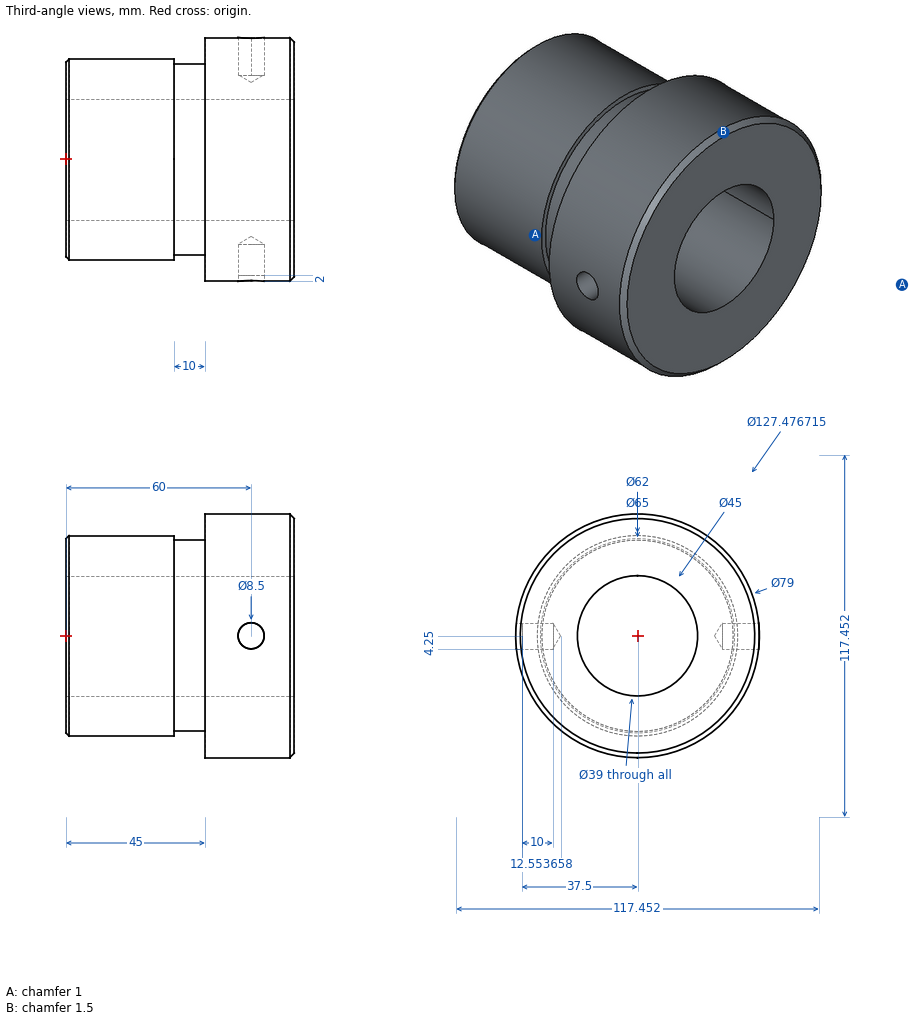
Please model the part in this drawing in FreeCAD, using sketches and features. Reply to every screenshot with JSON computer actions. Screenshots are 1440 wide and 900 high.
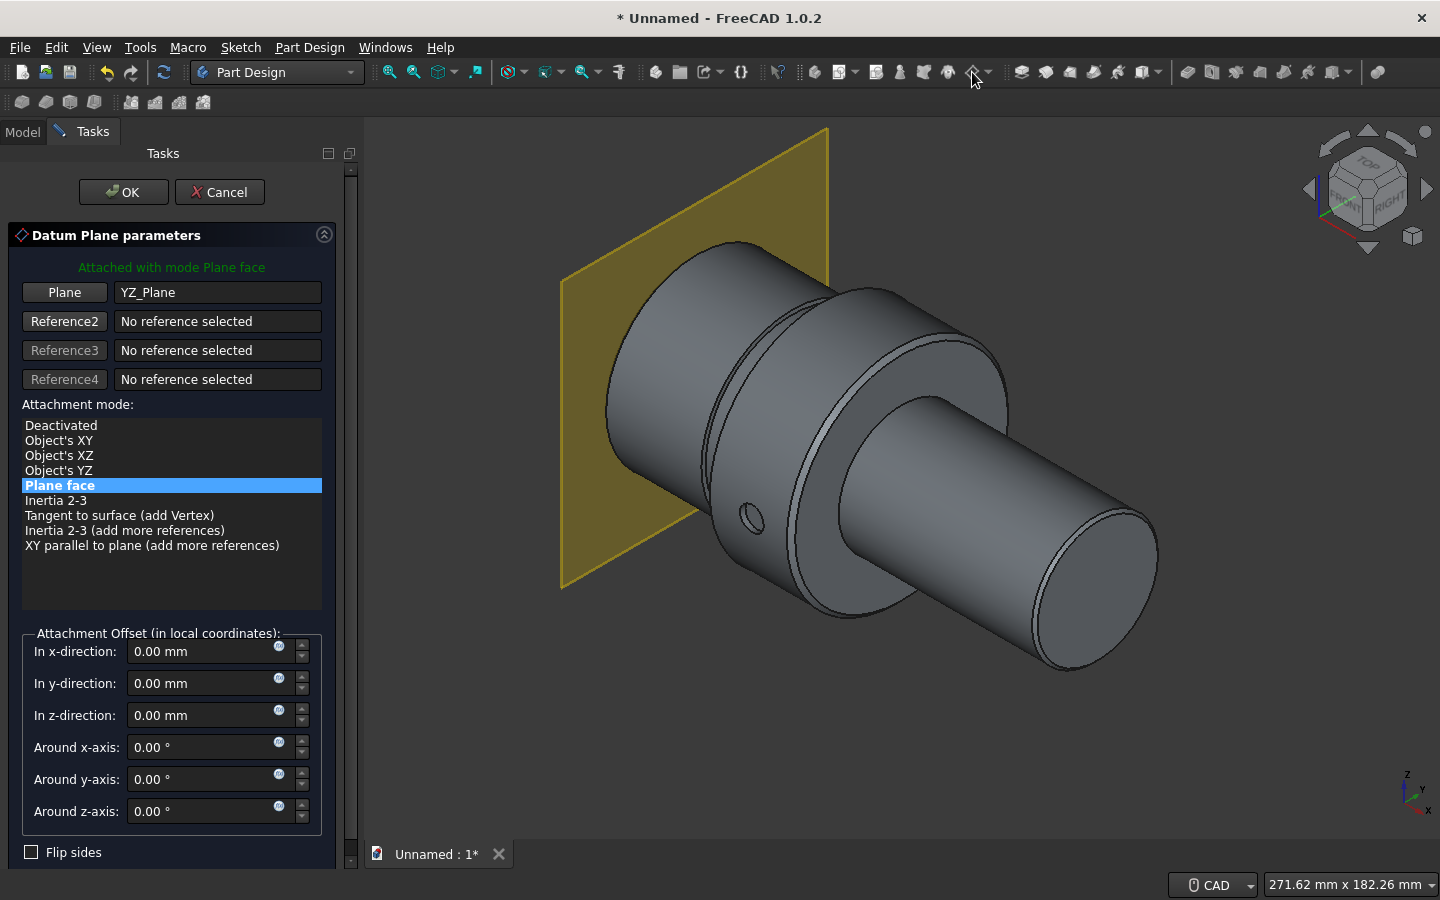
{"action": "triple_click", "coordinate": [210, 715]}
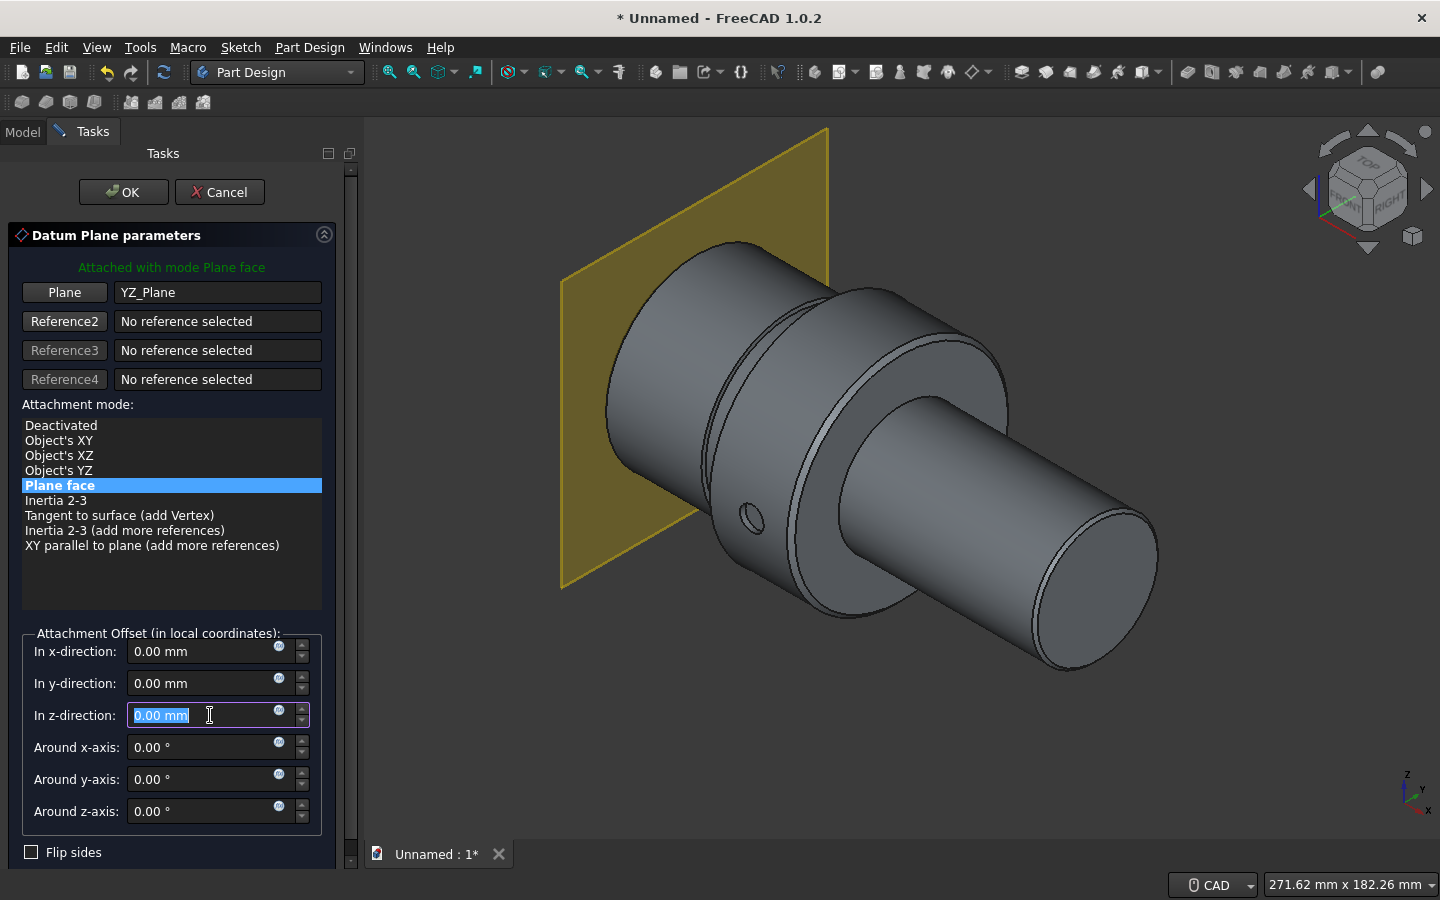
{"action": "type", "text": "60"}
{"action": "key", "text": "Tab"}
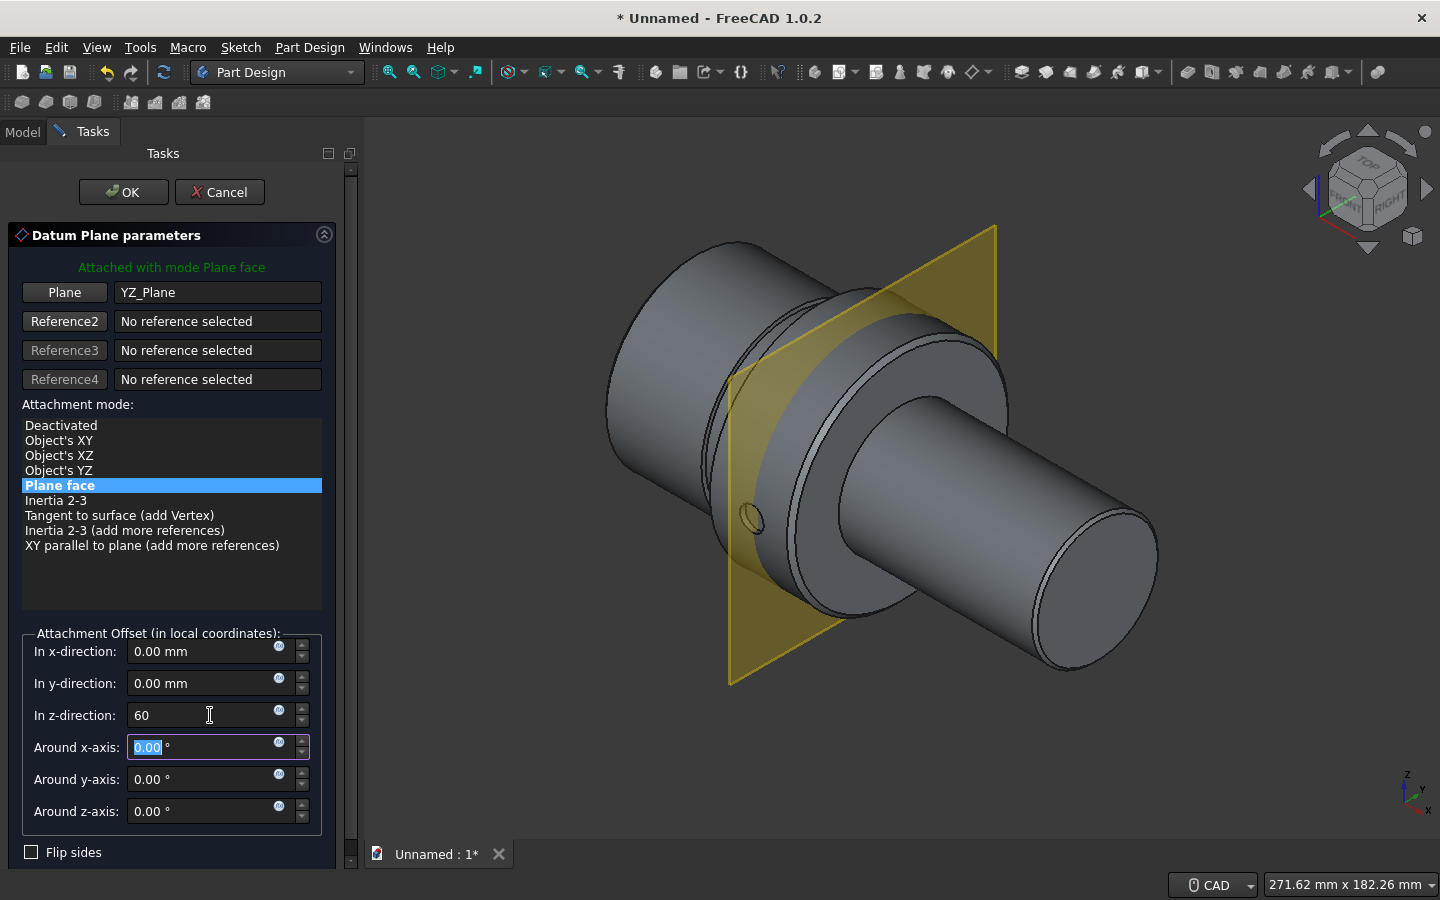
{"action": "left_click", "coordinate": [124, 192]}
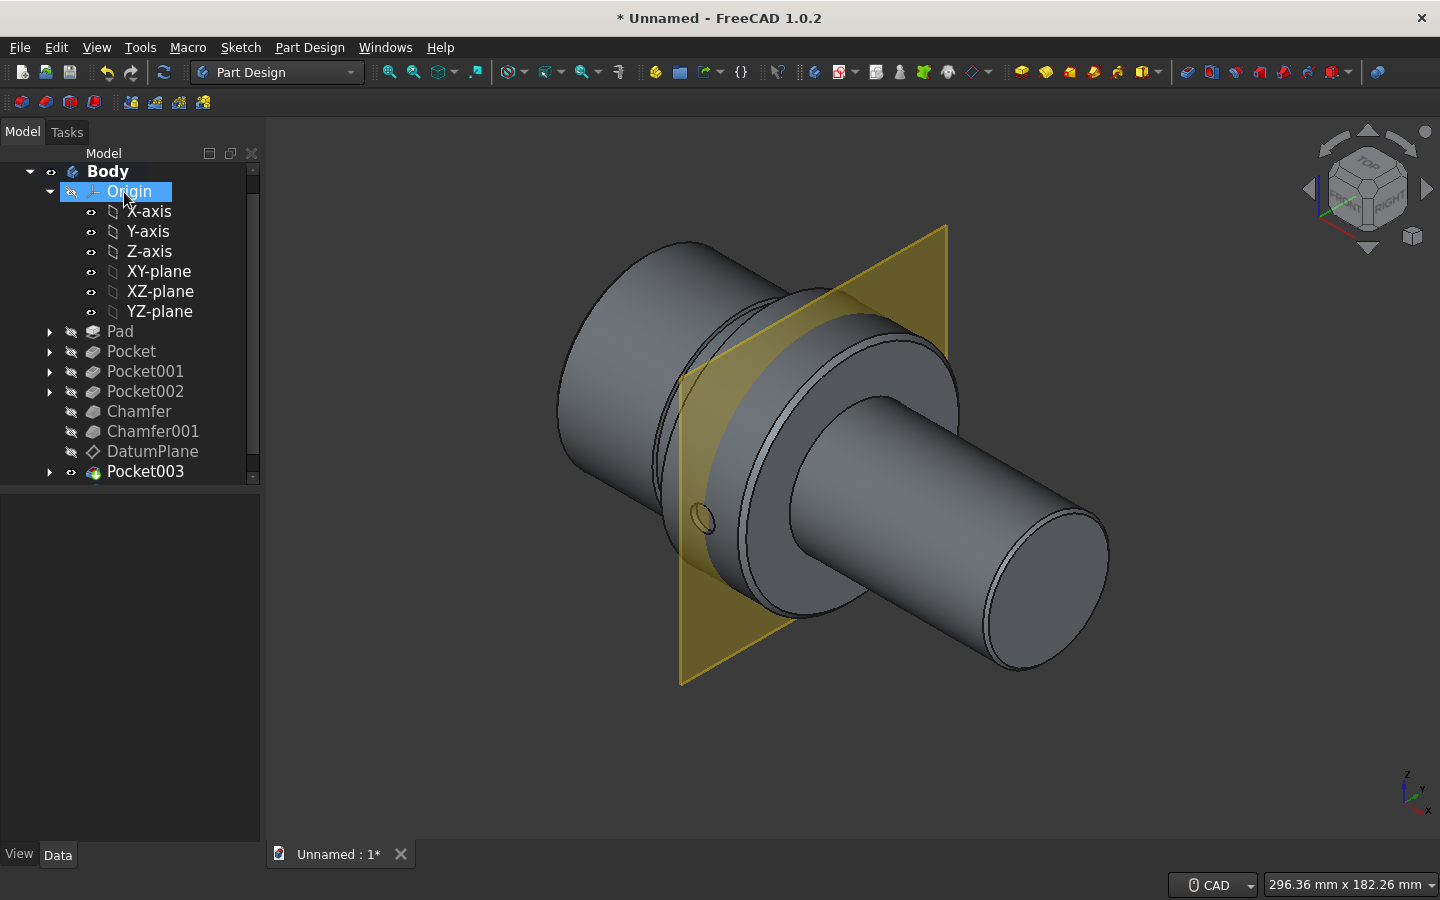
{"action": "scroll", "coordinate": [120, 327], "scroll_direction": "down", "scroll_amount": 3}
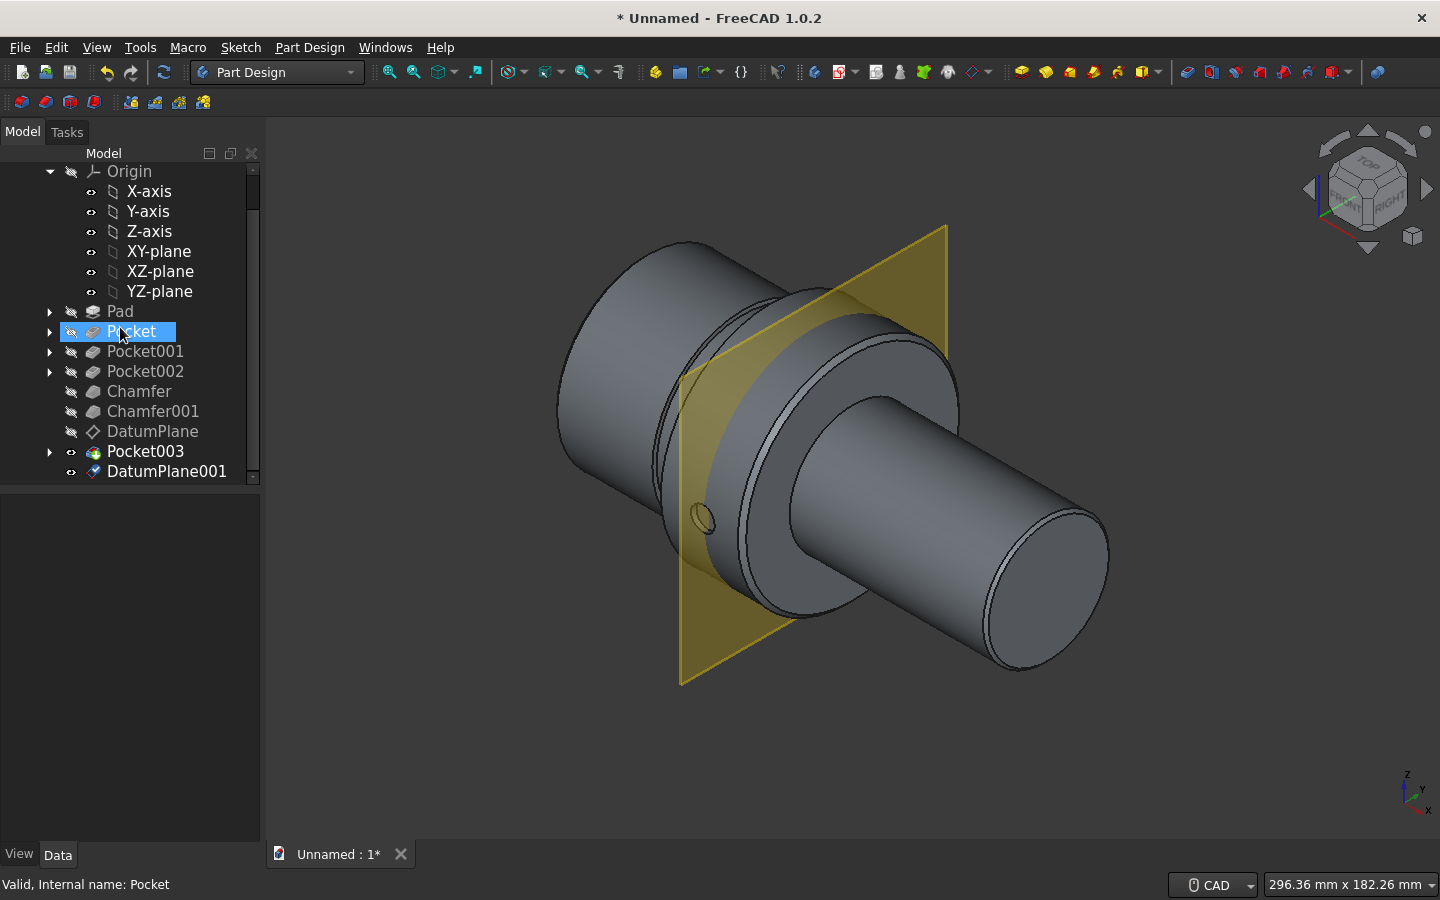
{"action": "left_click", "coordinate": [116, 472]}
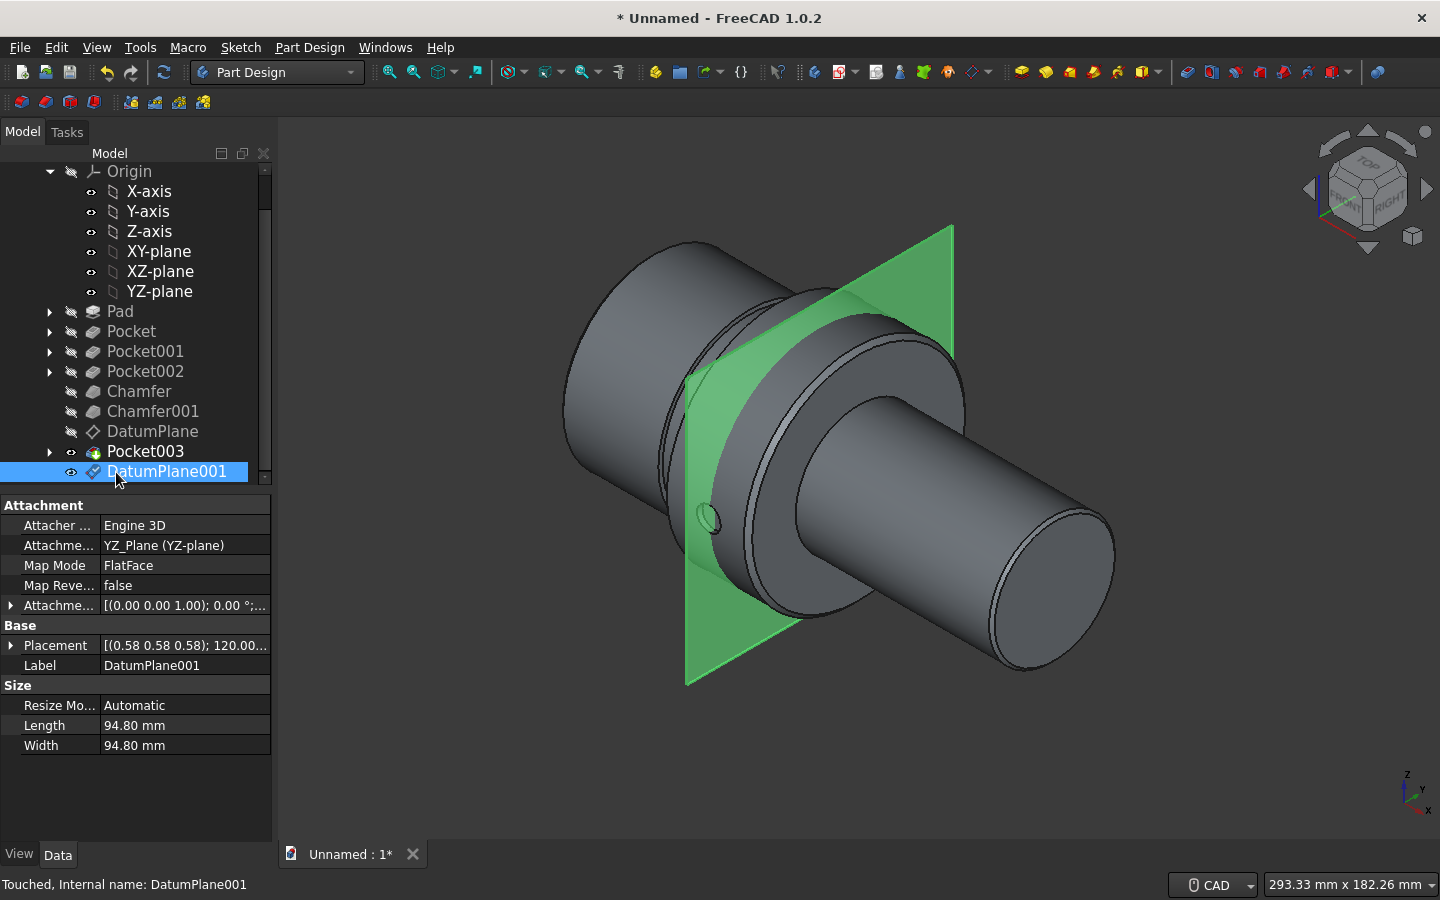
{"action": "left_click", "coordinate": [840, 72]}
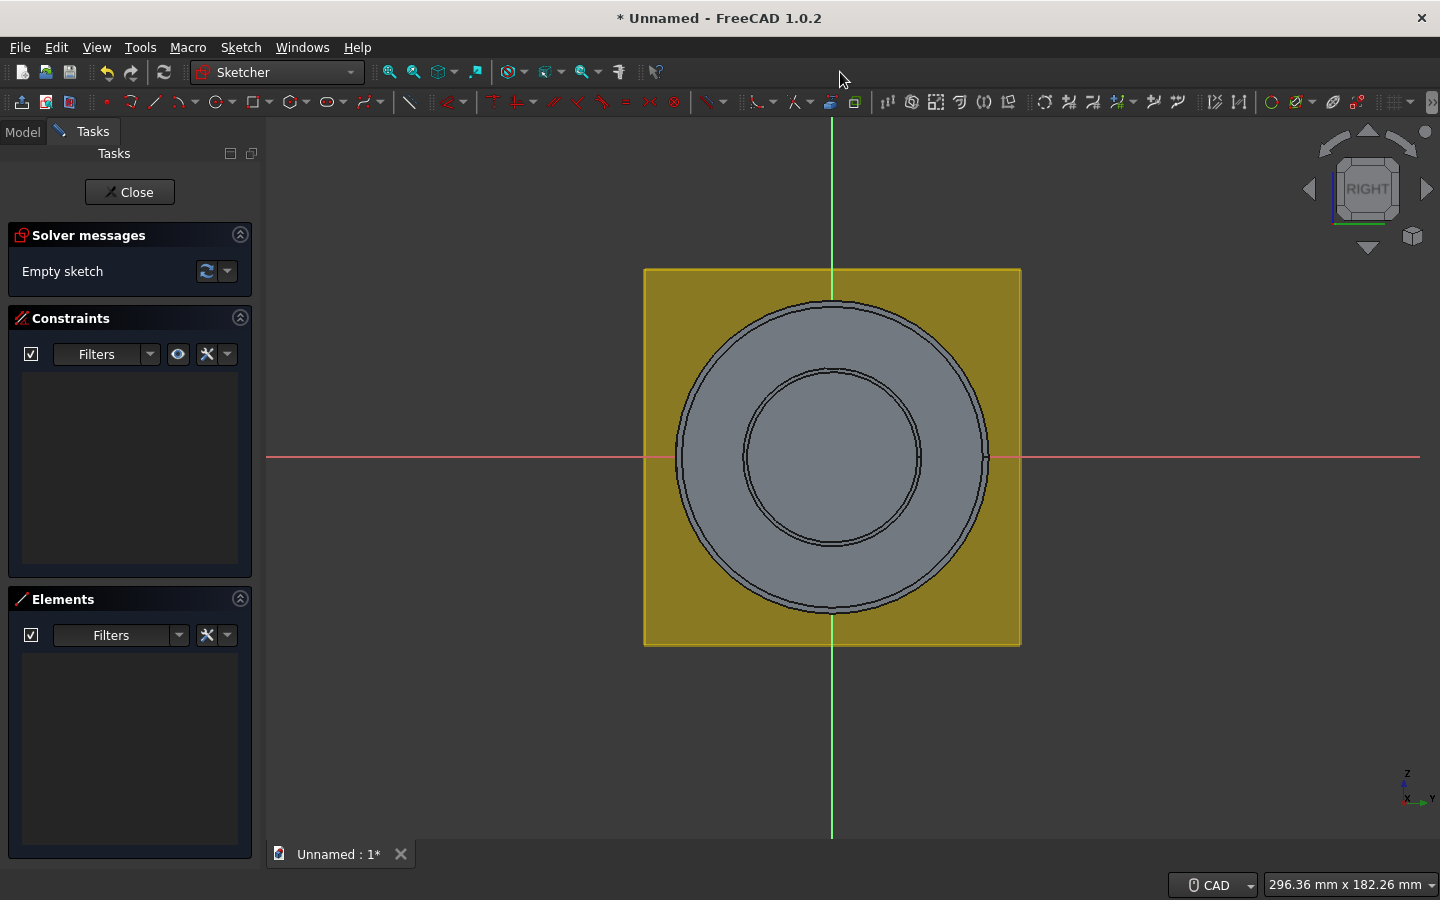
{"action": "key", "text": "q s"}